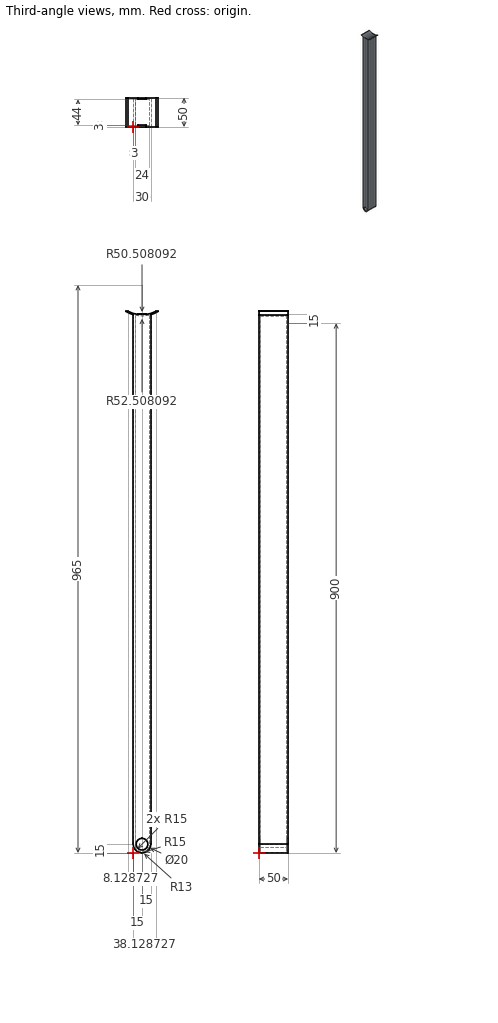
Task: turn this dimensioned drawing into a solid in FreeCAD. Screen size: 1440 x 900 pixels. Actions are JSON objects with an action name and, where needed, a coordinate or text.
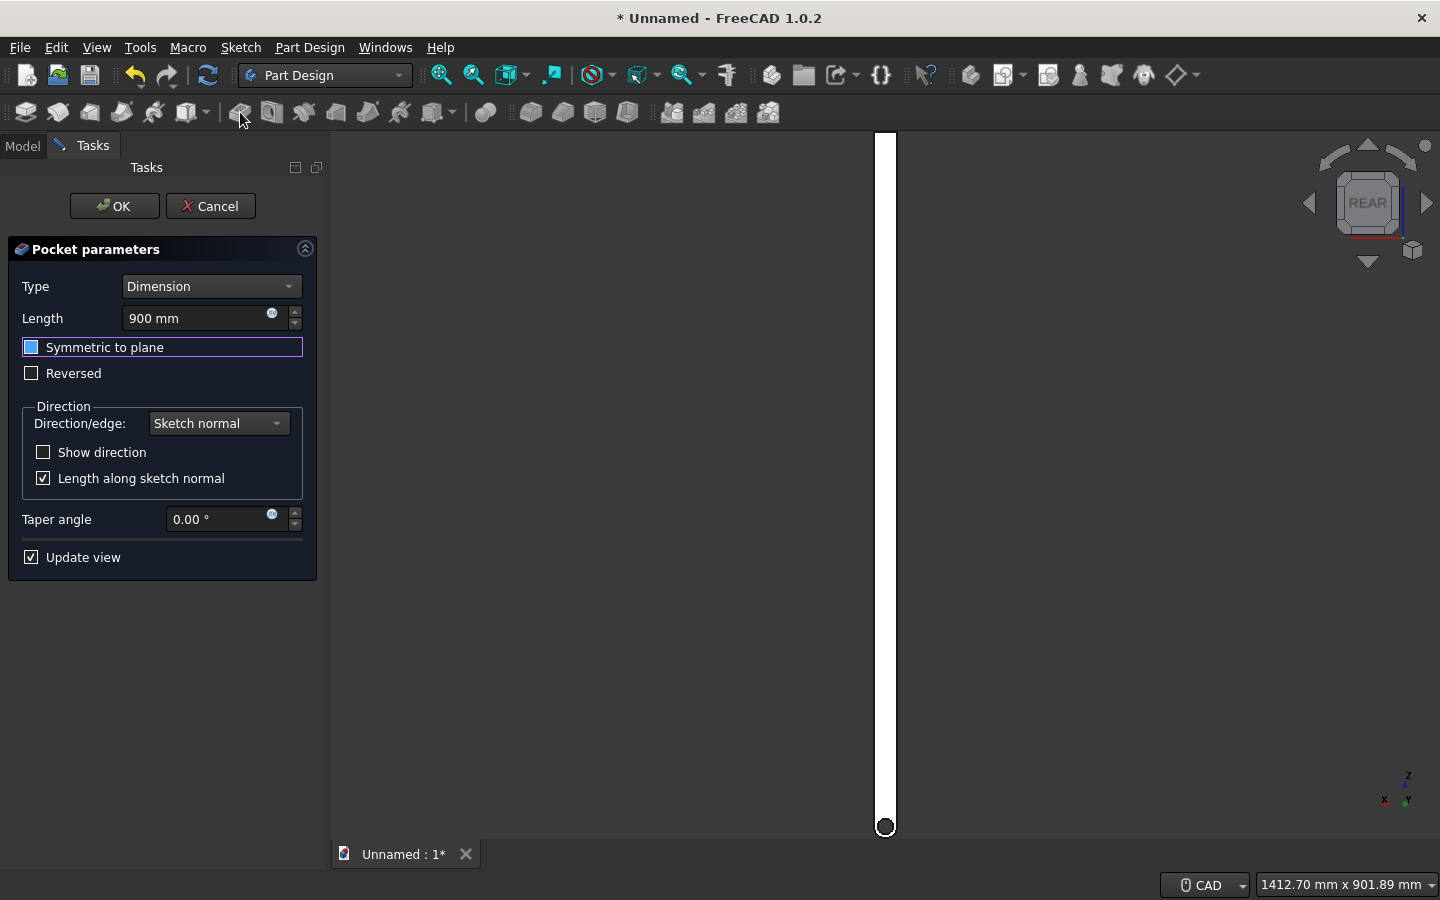
{"action": "left_click", "coordinate": [115, 206]}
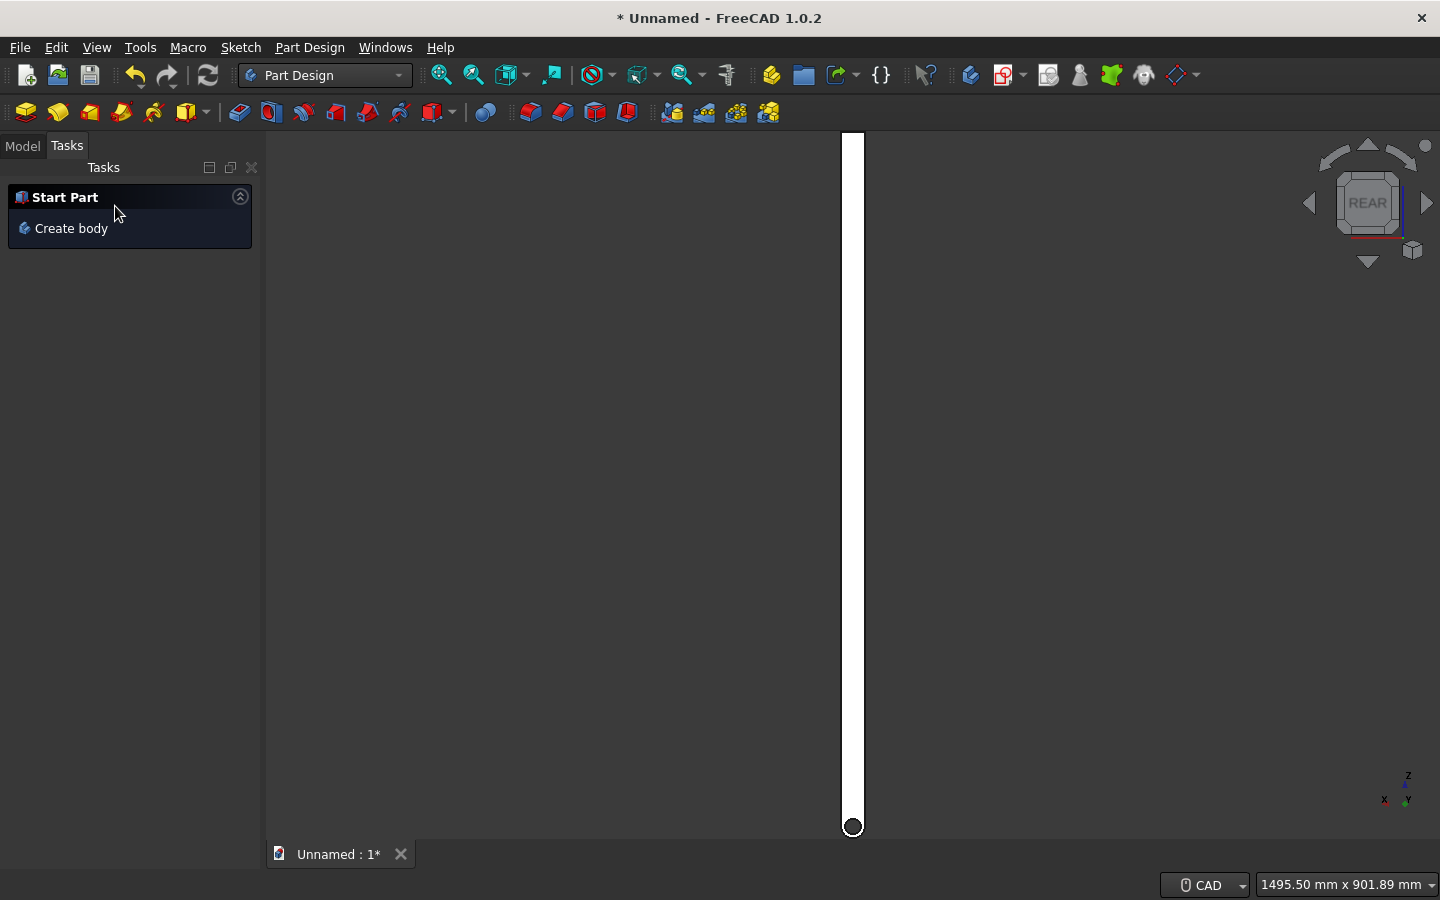
{"action": "left_click", "coordinate": [853, 181]}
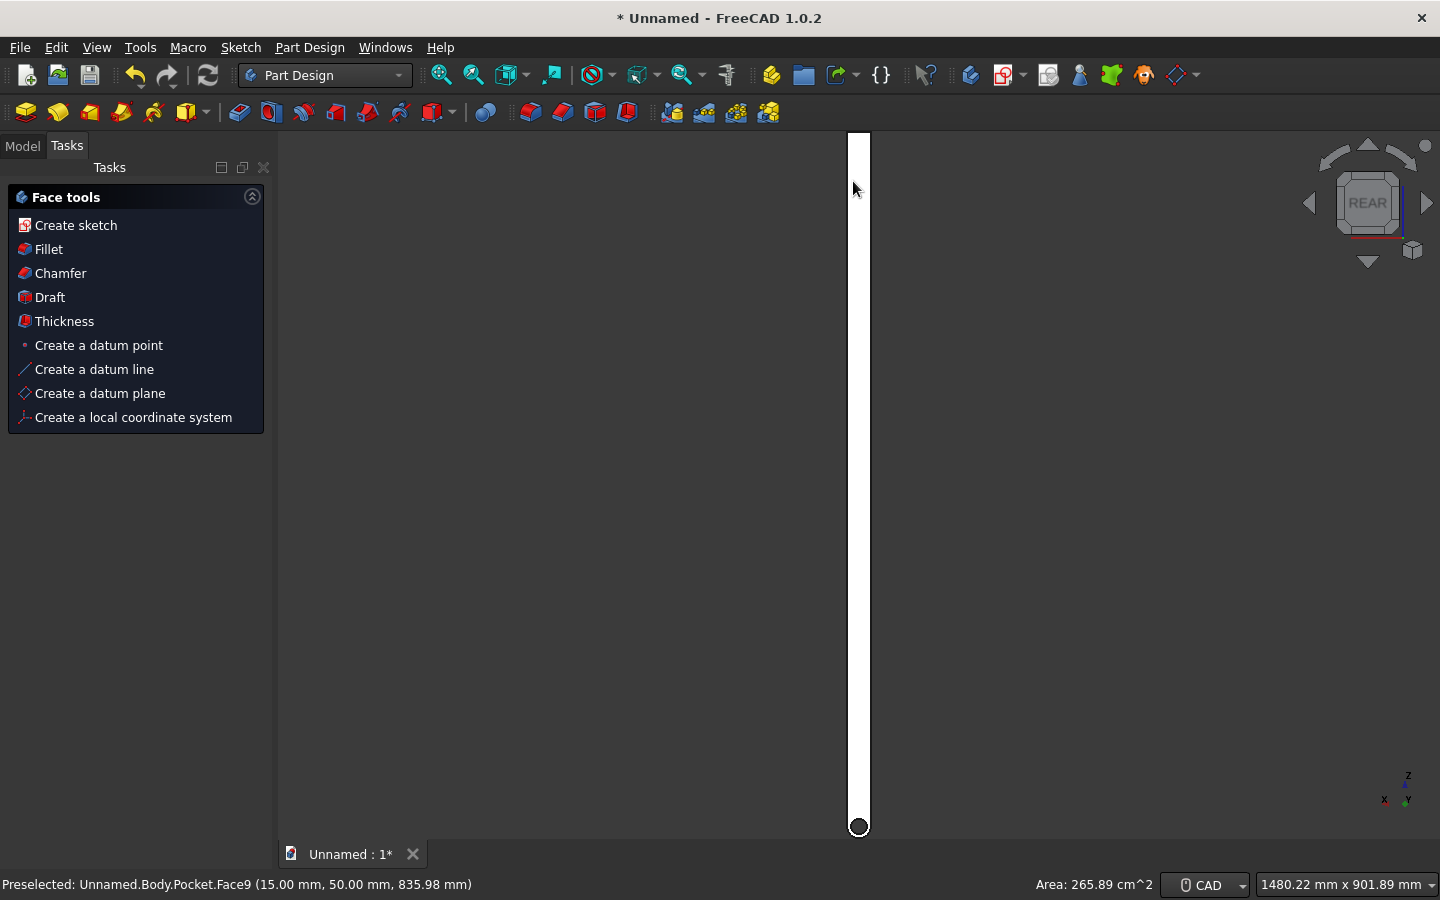
{"action": "left_click", "coordinate": [1004, 76]}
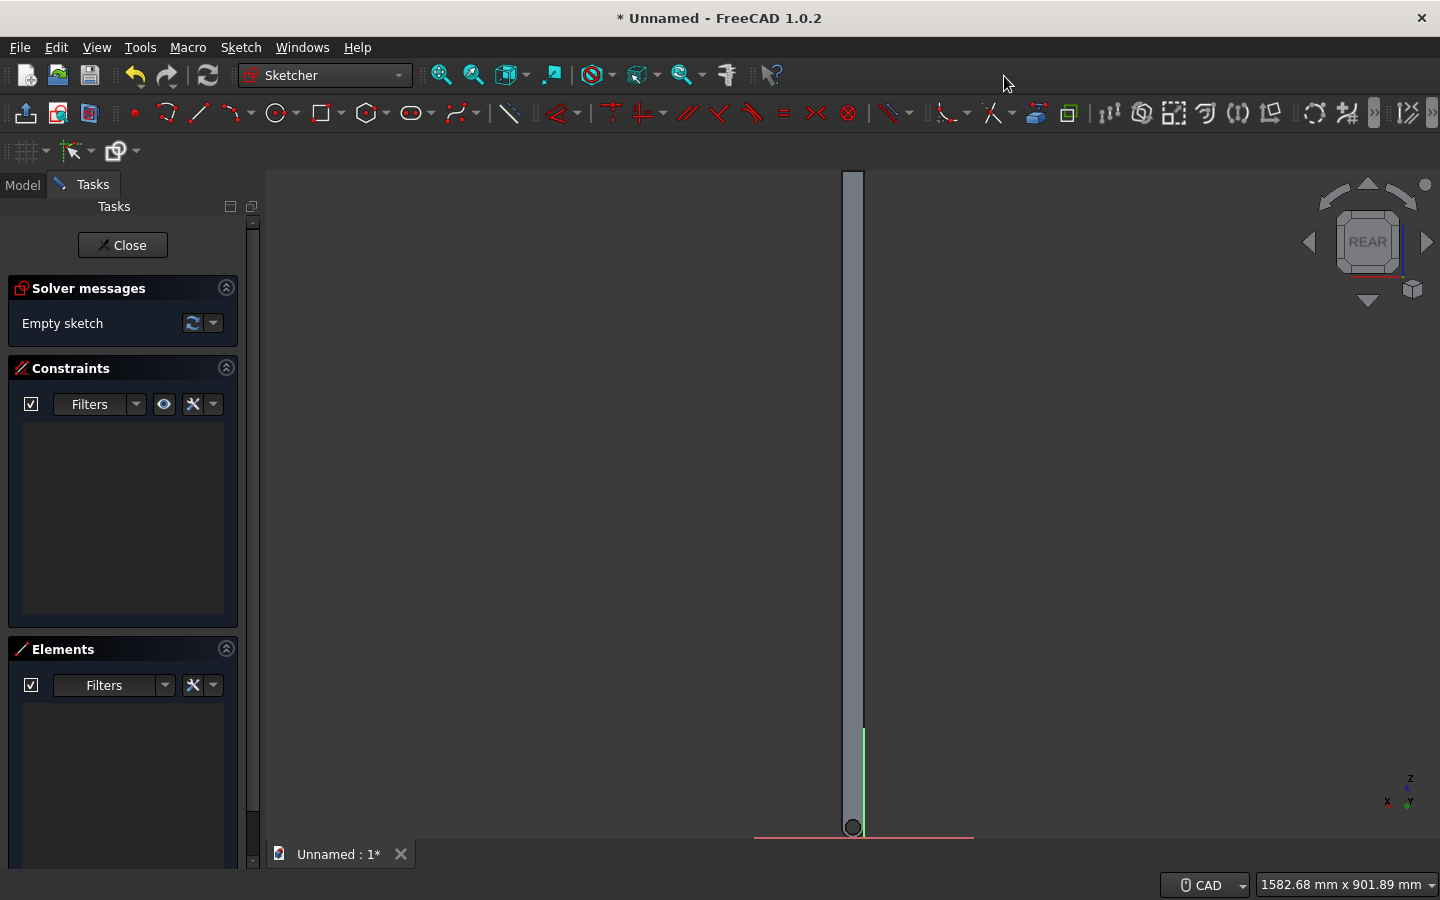
{"action": "scroll", "coordinate": [784, 504], "scroll_direction": "down", "scroll_amount": 5}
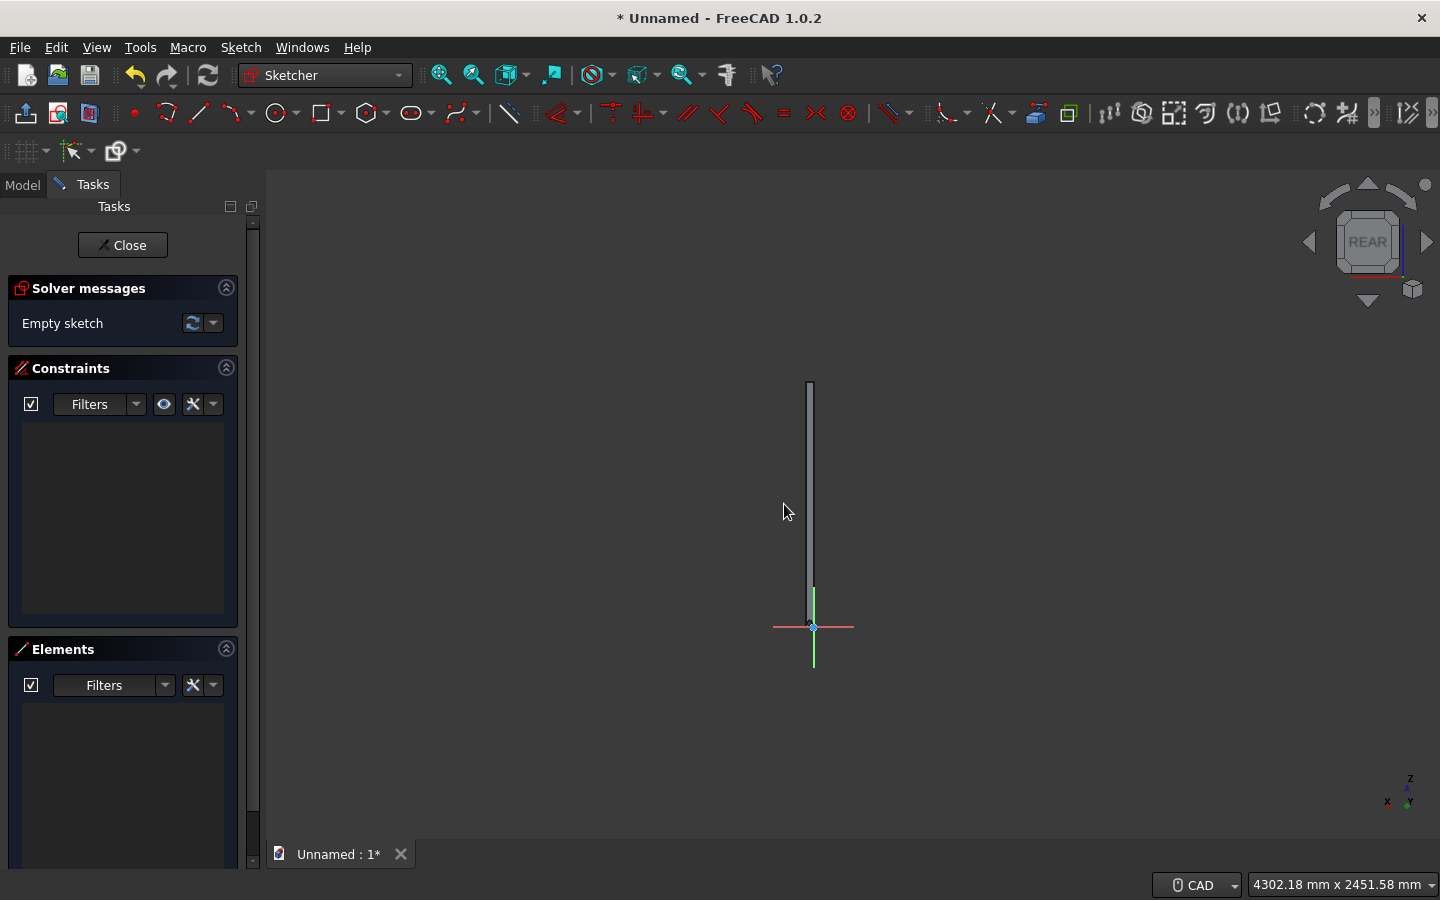
{"action": "scroll", "coordinate": [811, 632], "scroll_direction": "up", "scroll_amount": 15}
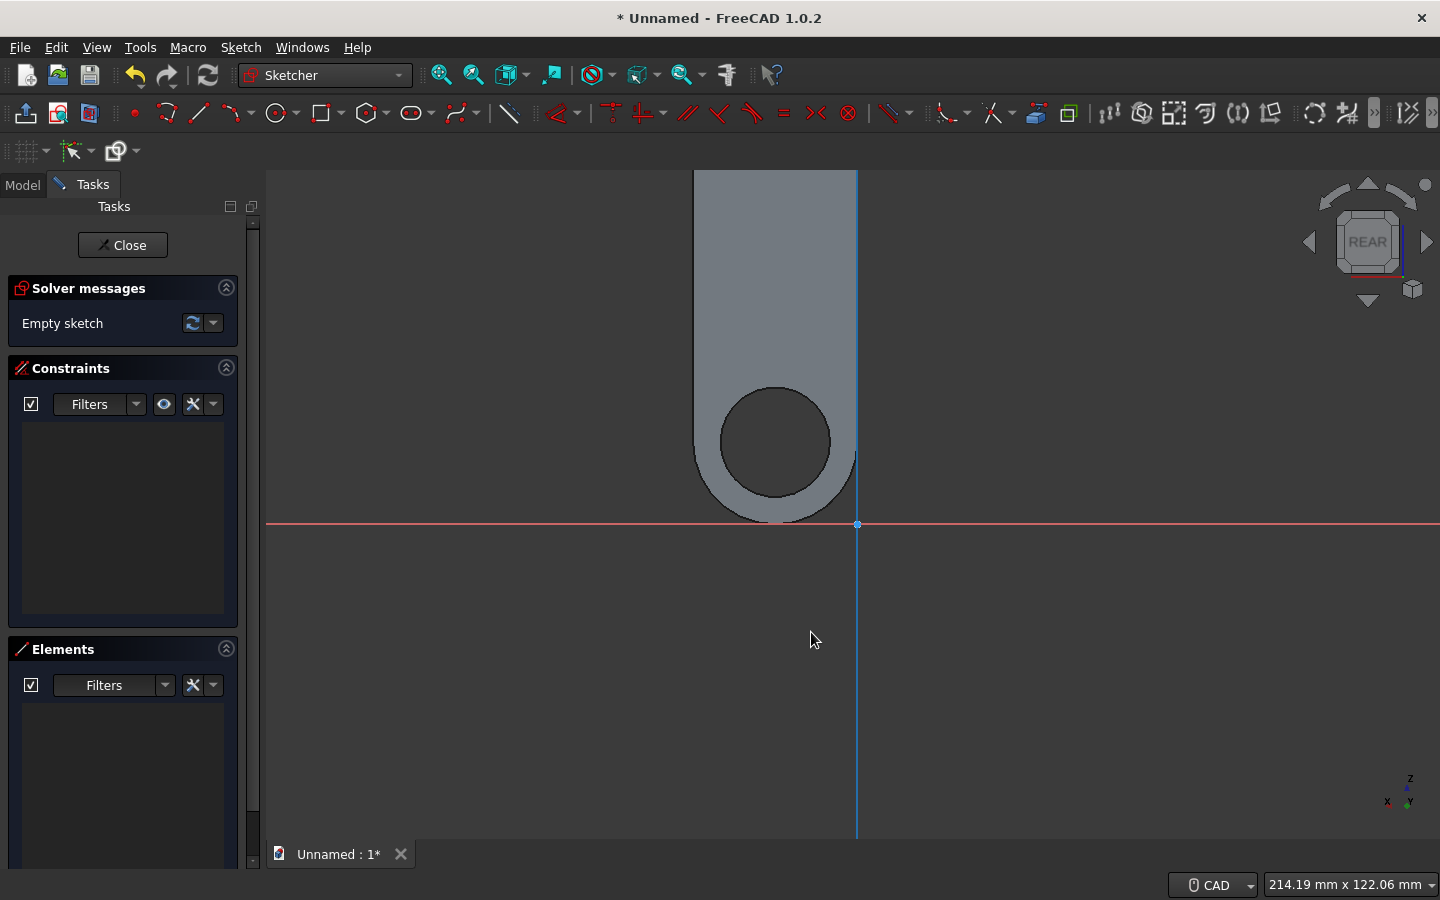
{"action": "scroll", "coordinate": [772, 476], "scroll_direction": "up", "scroll_amount": 7}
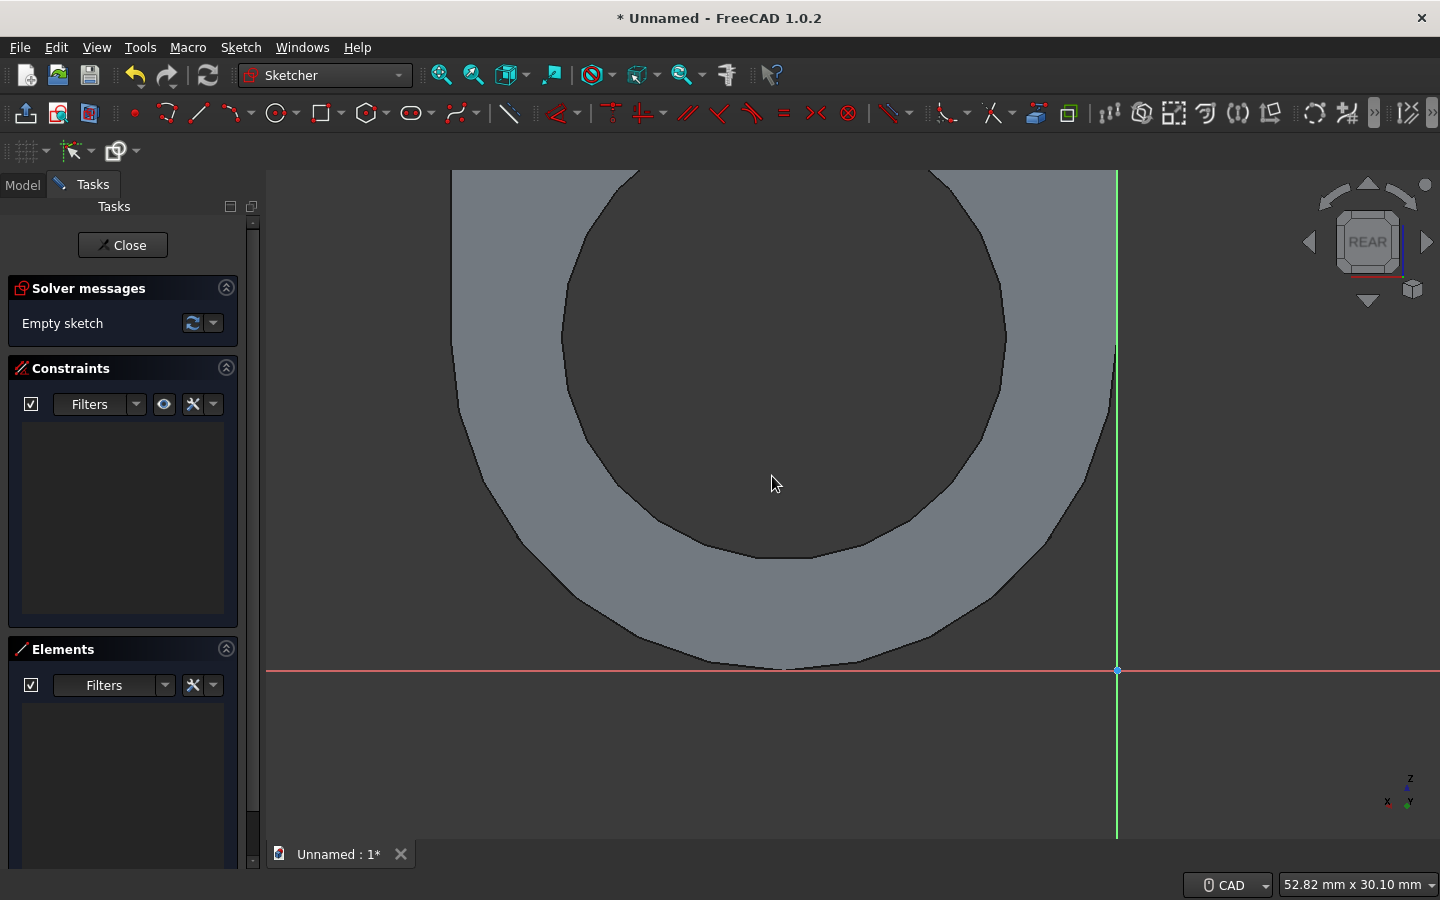
{"action": "left_click", "coordinate": [200, 114]}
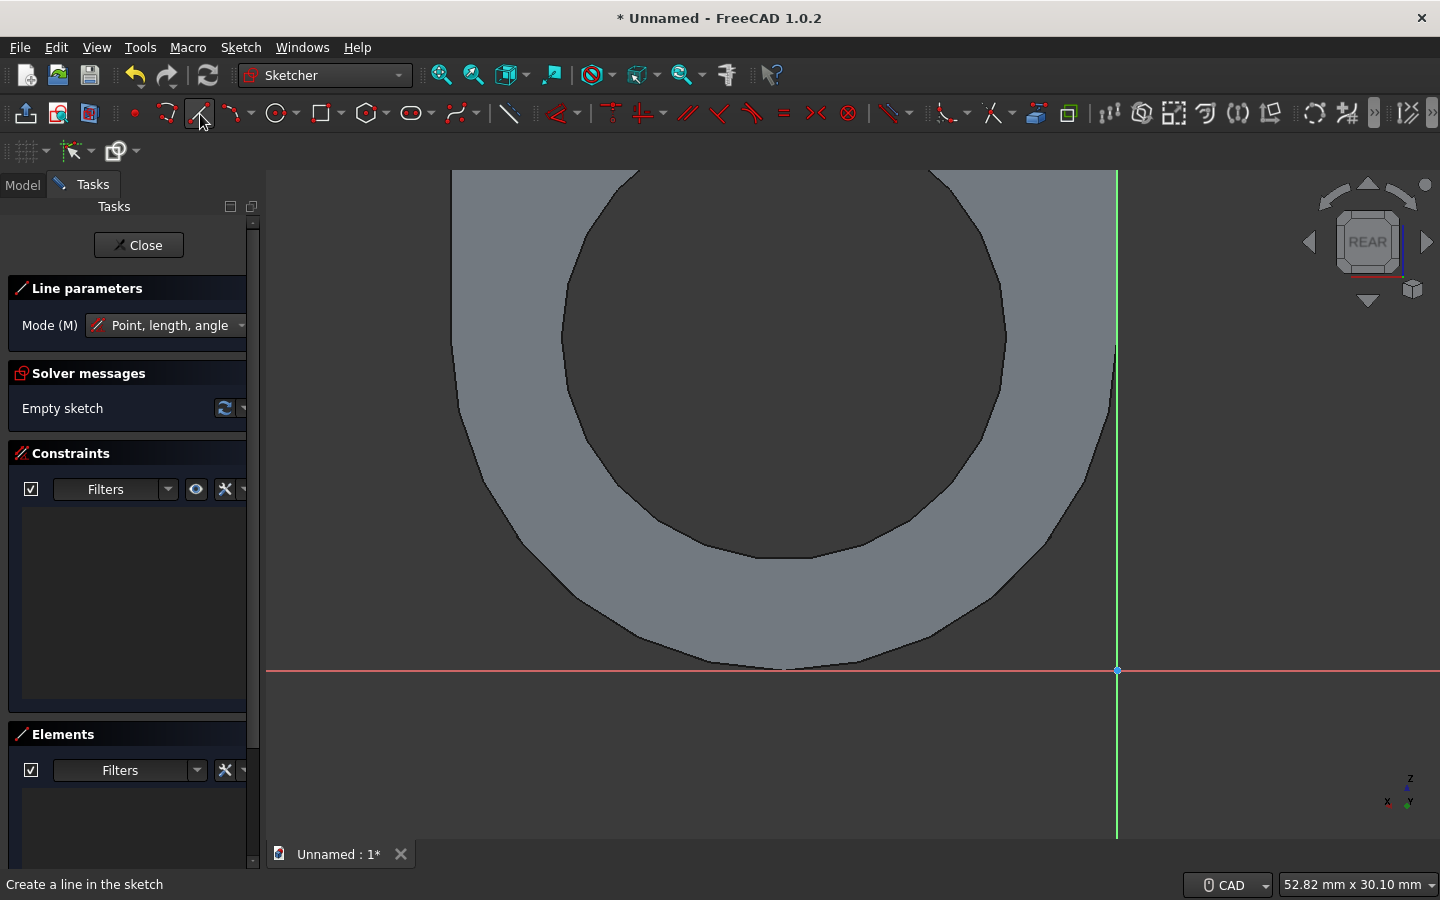
{"action": "left_click", "coordinate": [1117, 337]}
{"action": "left_click", "coordinate": [1073, 337]}